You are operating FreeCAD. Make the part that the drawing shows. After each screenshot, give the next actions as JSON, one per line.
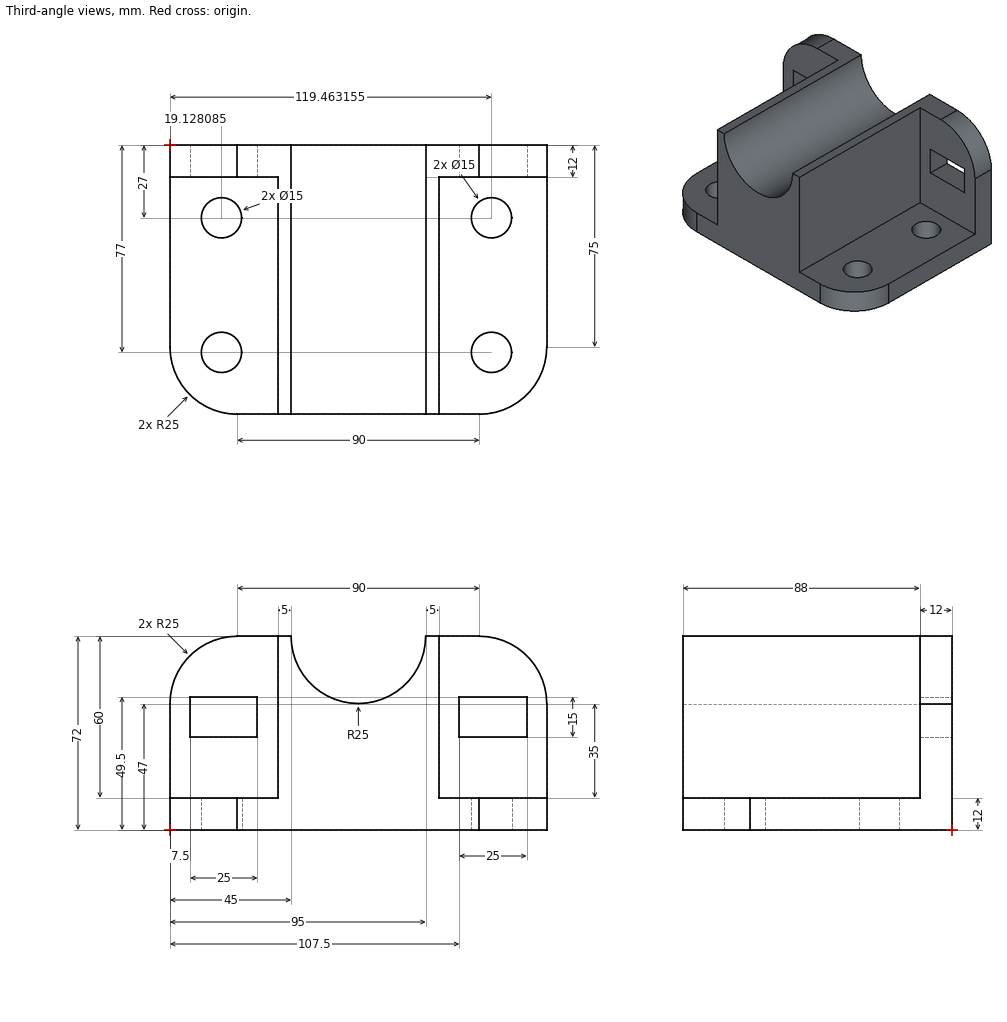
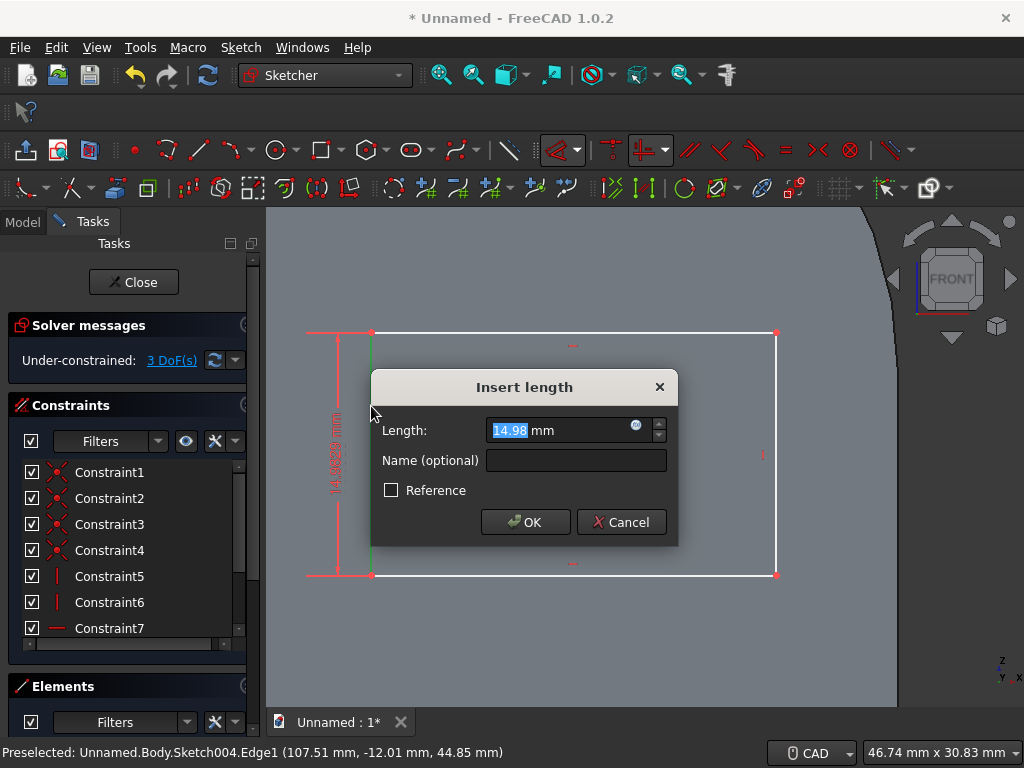
{"action": "type", "text": "15"}
{"action": "key", "text": "Return"}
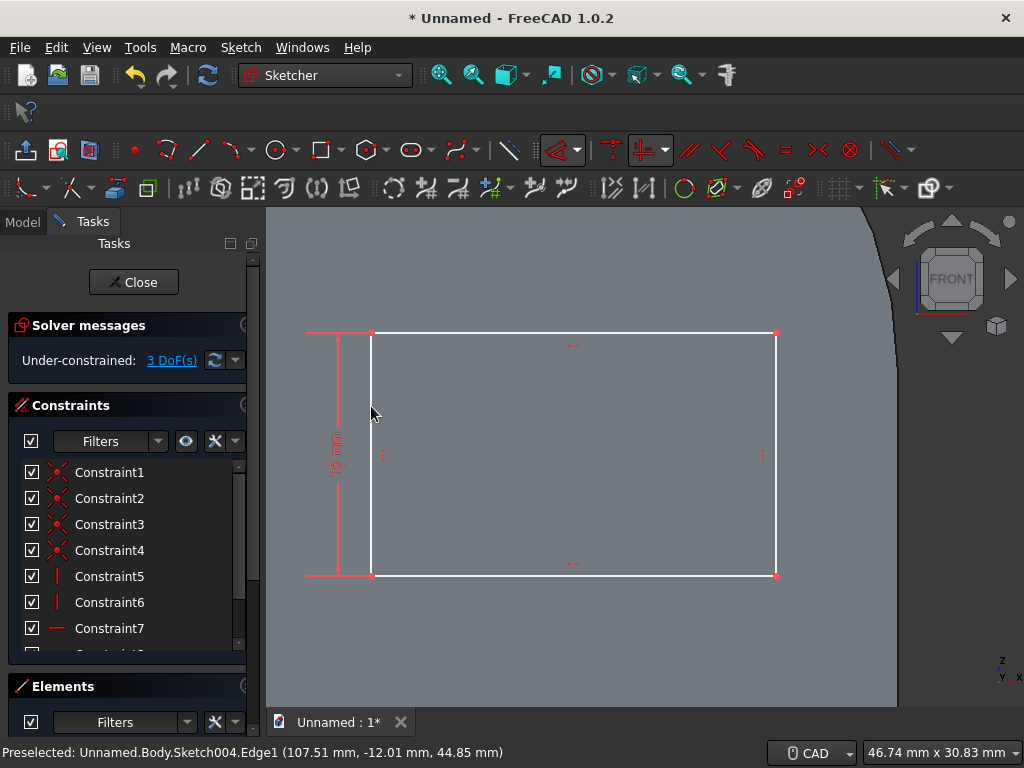
{"action": "left_click", "coordinate": [493, 576]}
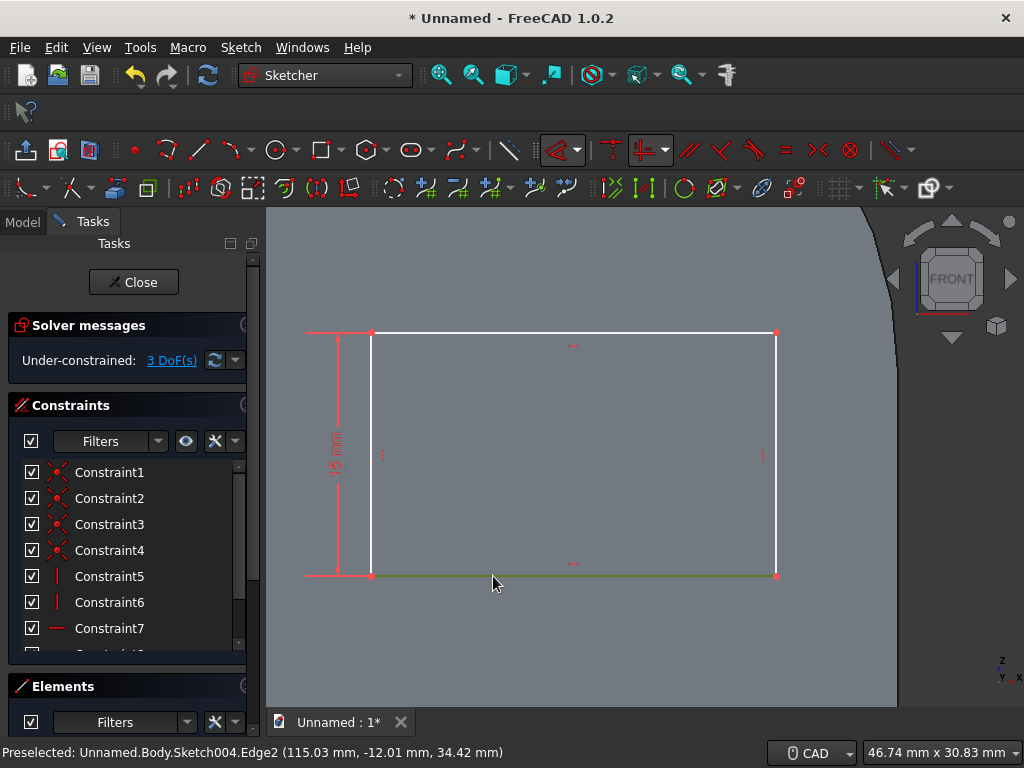
{"action": "key", "text": "l"}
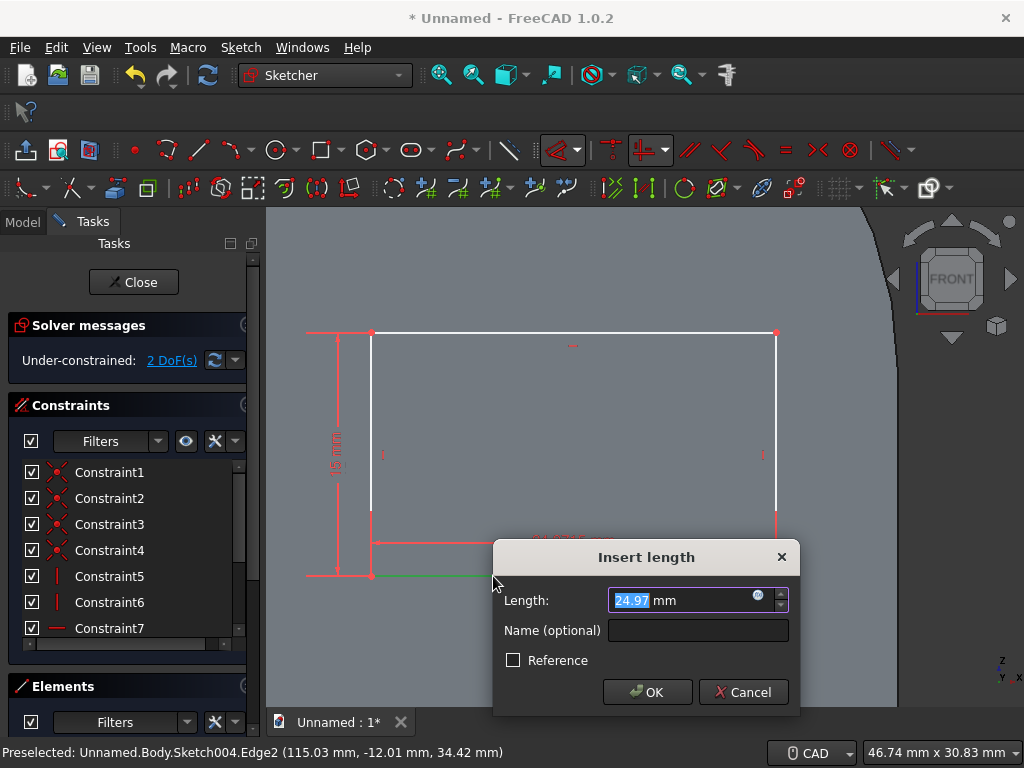
{"action": "type", "text": "25"}
{"action": "key", "text": "Return"}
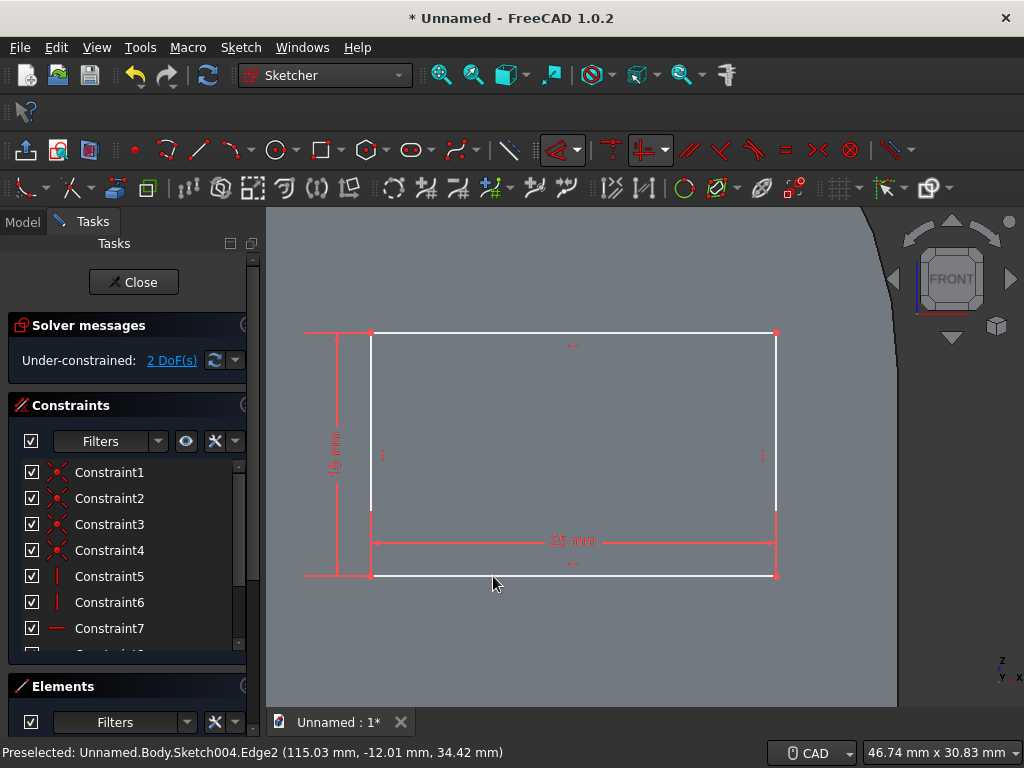
{"action": "left_click", "coordinate": [371, 333]}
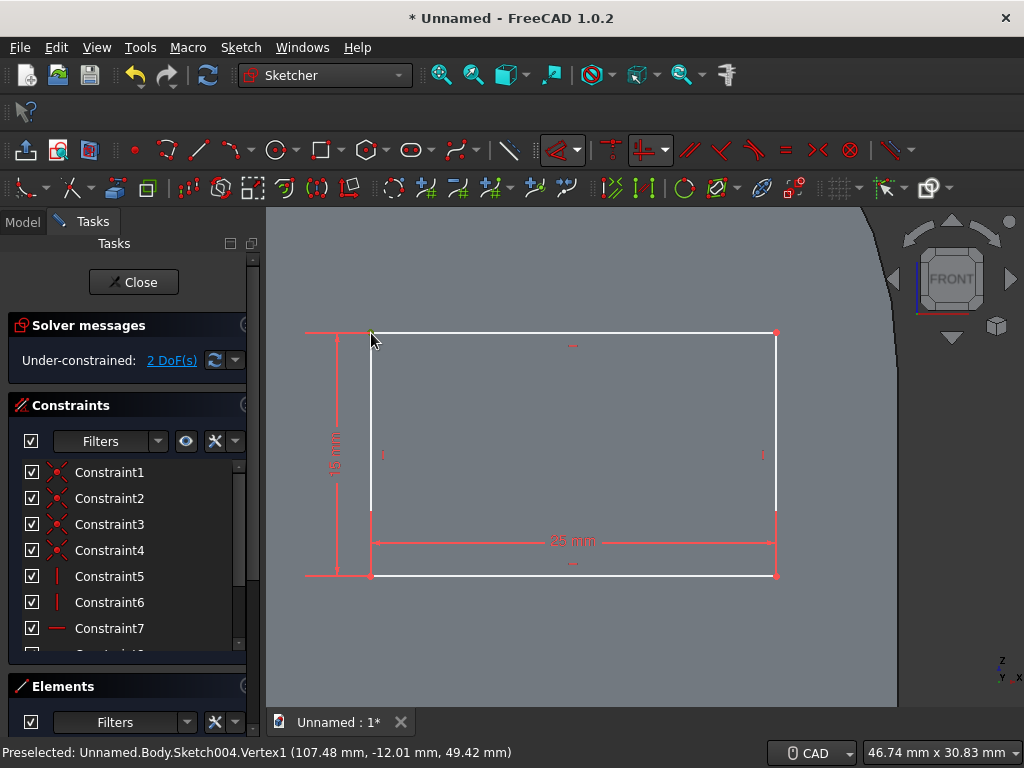
{"action": "key", "text": "i"}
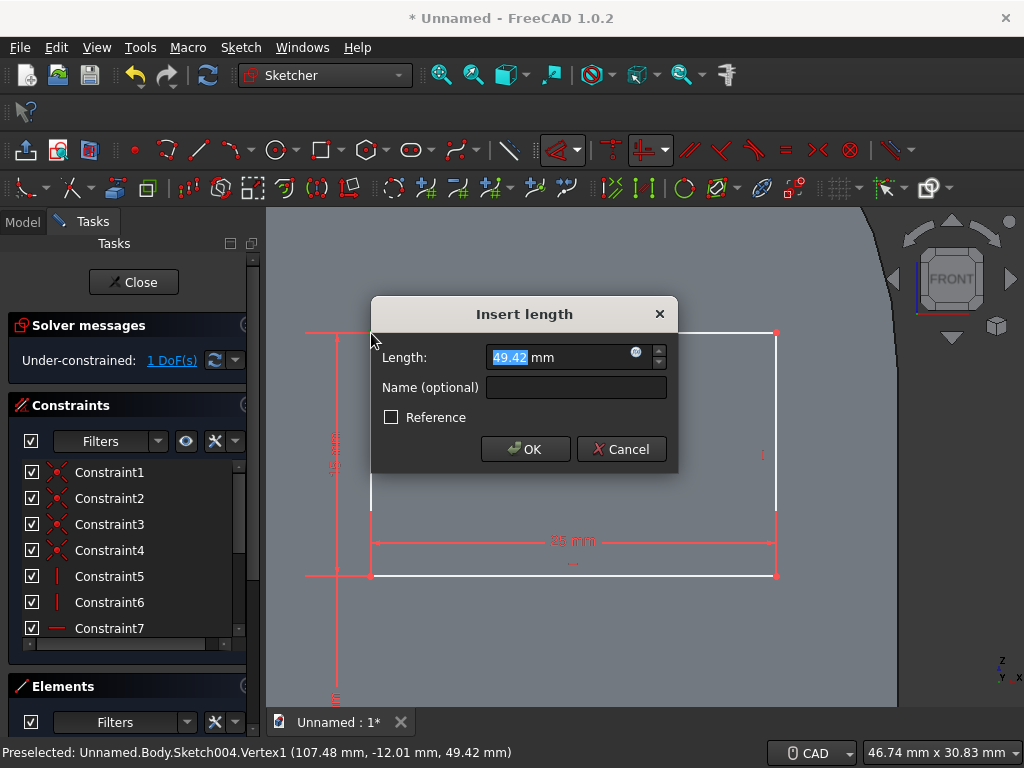
{"action": "type", "text": "49.5"}
{"action": "key", "text": "Return"}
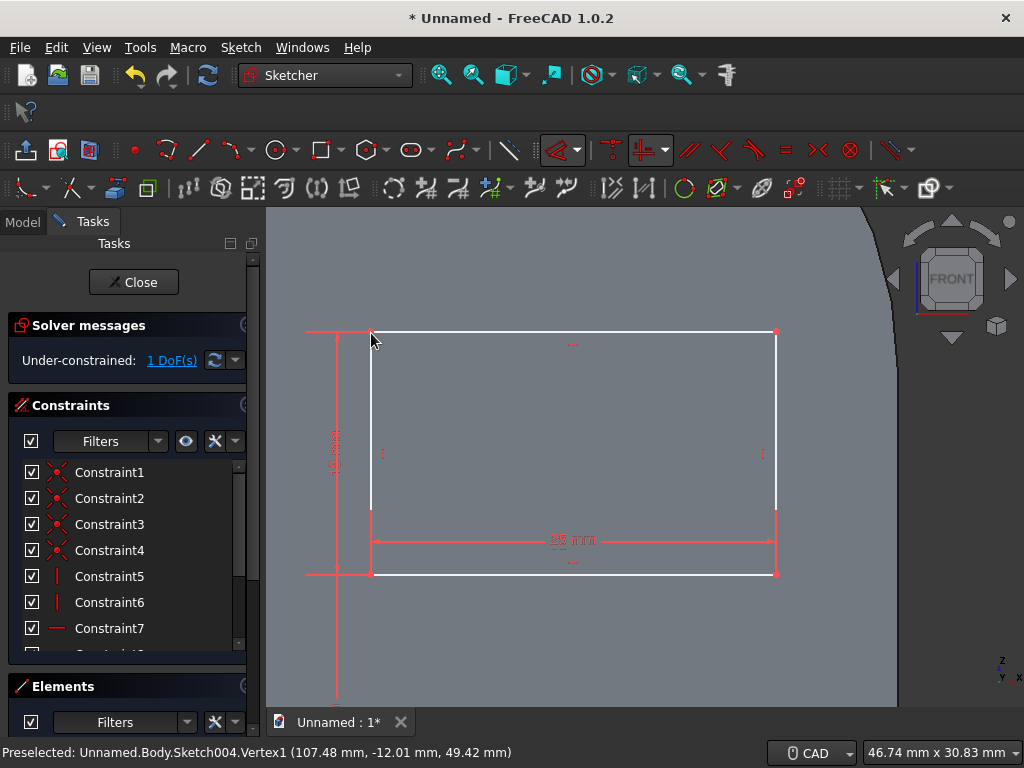
{"action": "left_click", "coordinate": [371, 332]}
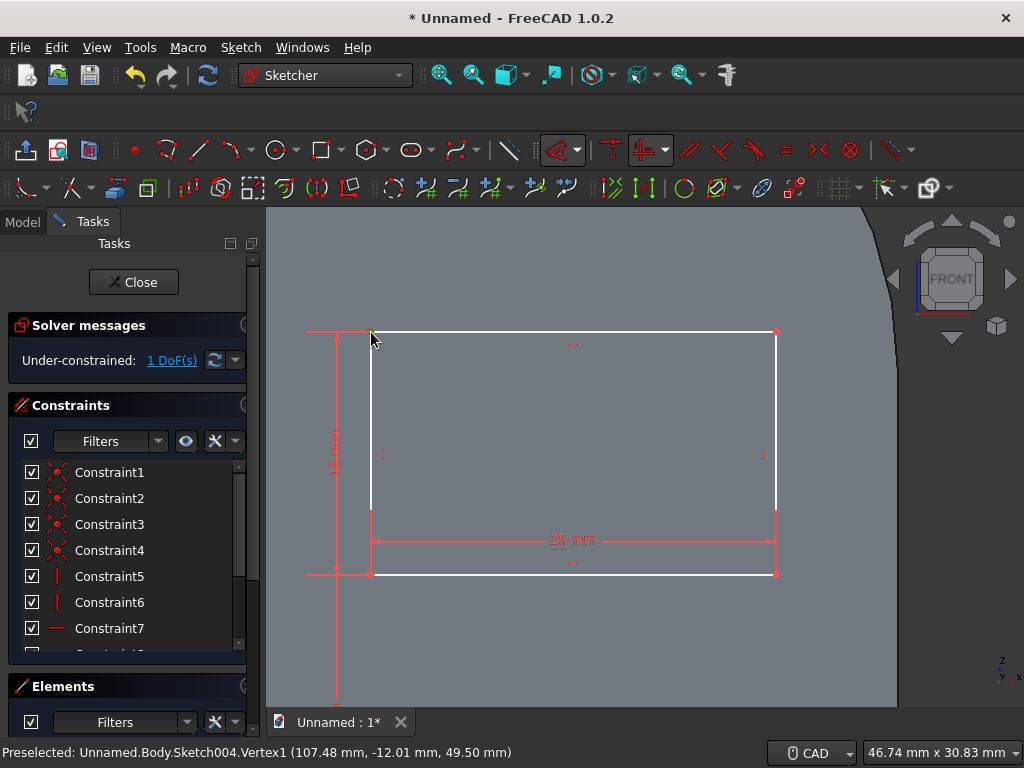
{"action": "key", "text": "l"}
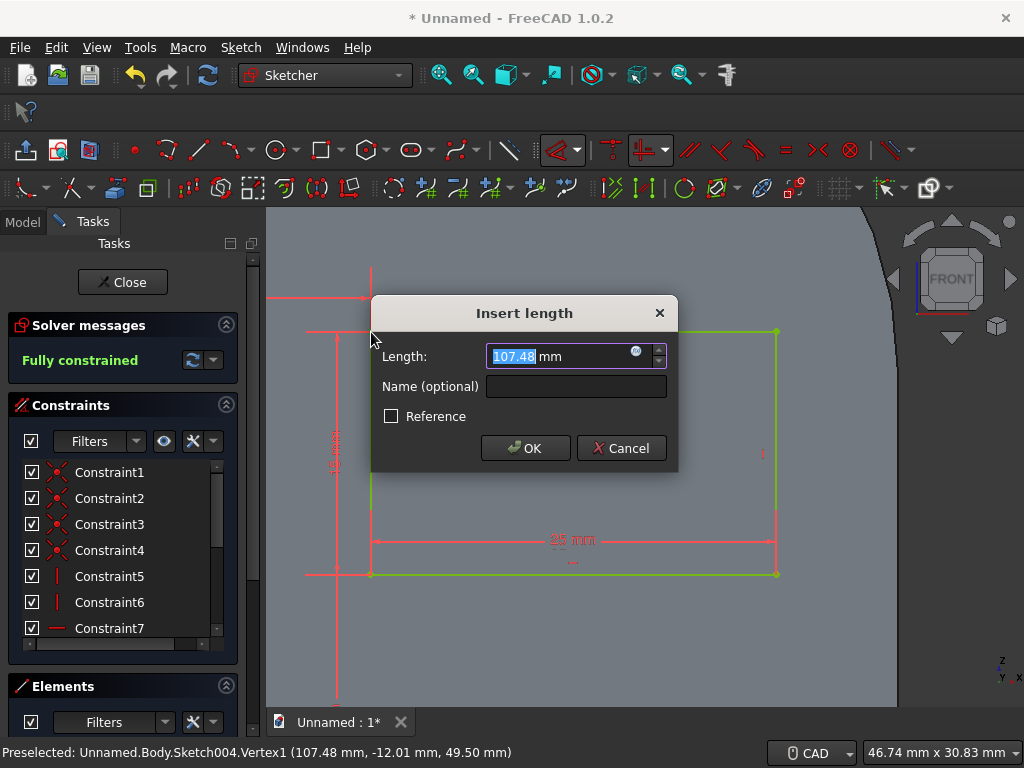
{"action": "type", "text": "107.5"}
{"action": "key", "text": "Return"}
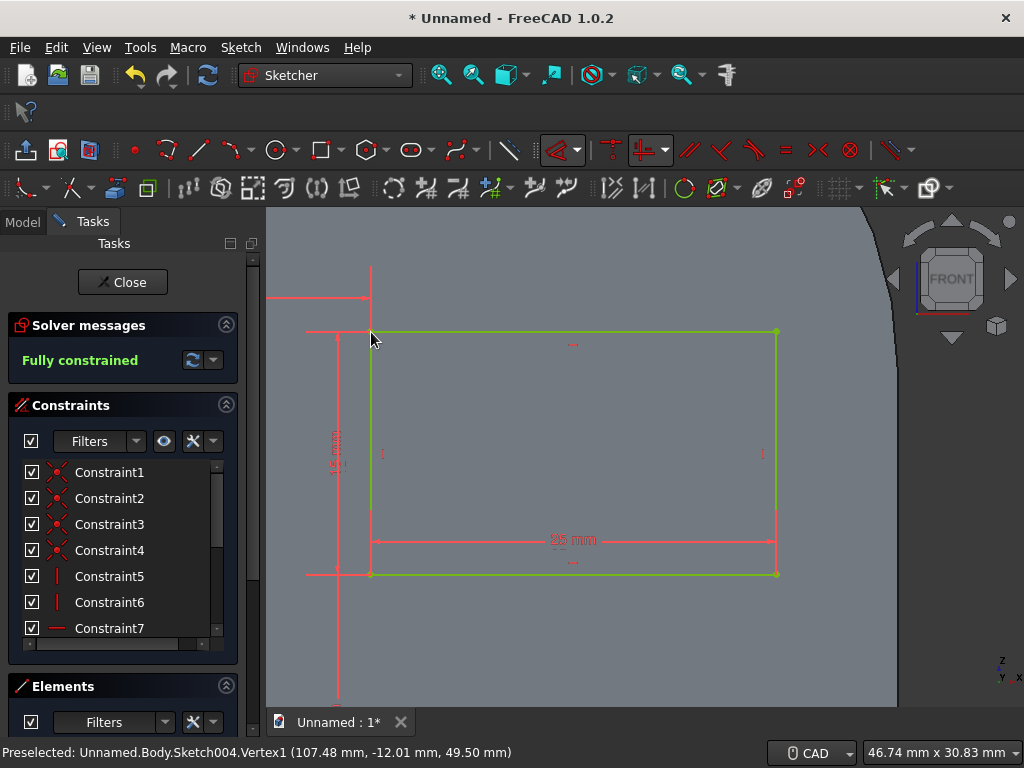
{"action": "left_click", "coordinate": [123, 282]}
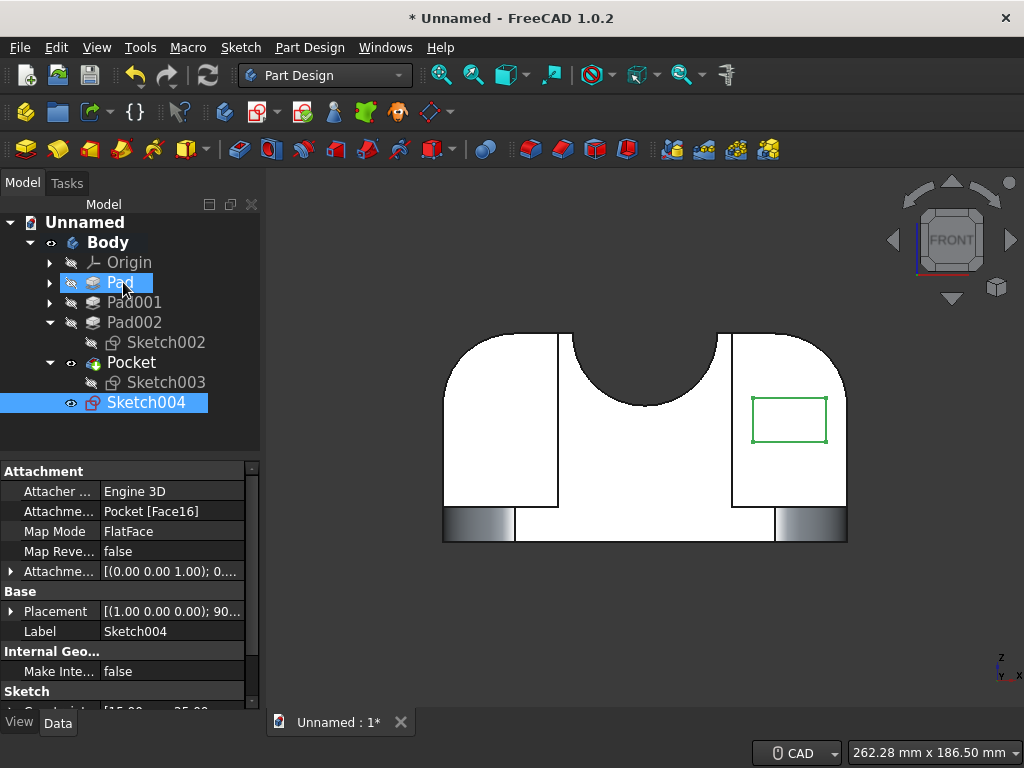
{"action": "left_click", "coordinate": [240, 150]}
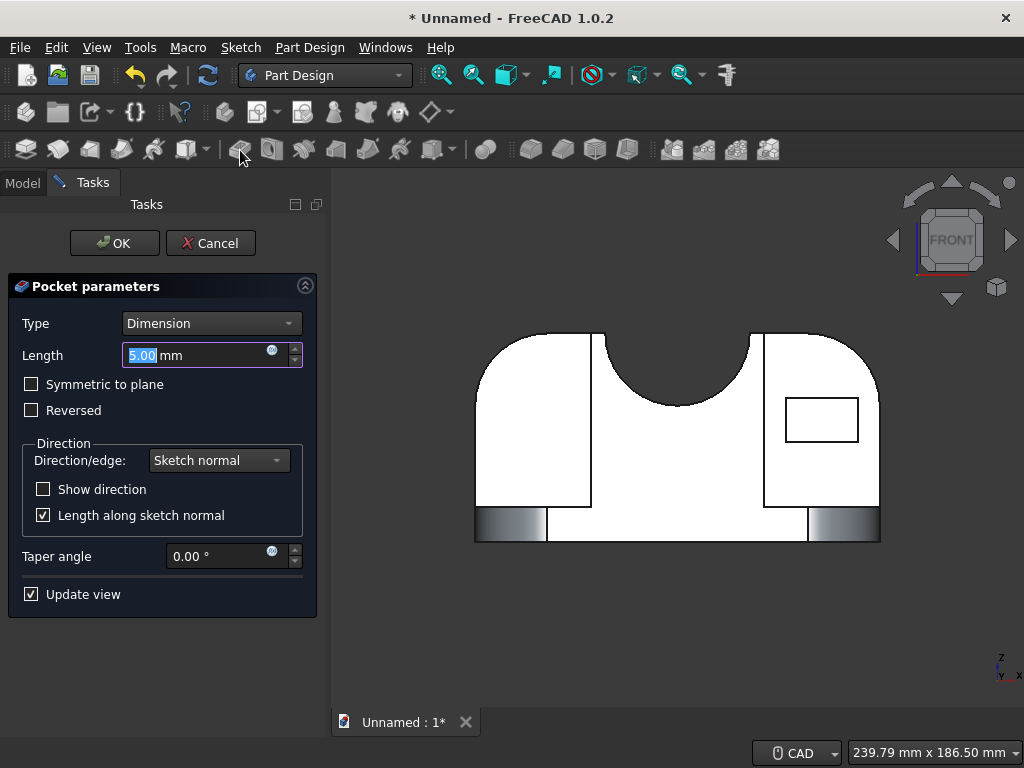
{"action": "type", "text": "12"}
{"action": "key", "text": "Tab"}